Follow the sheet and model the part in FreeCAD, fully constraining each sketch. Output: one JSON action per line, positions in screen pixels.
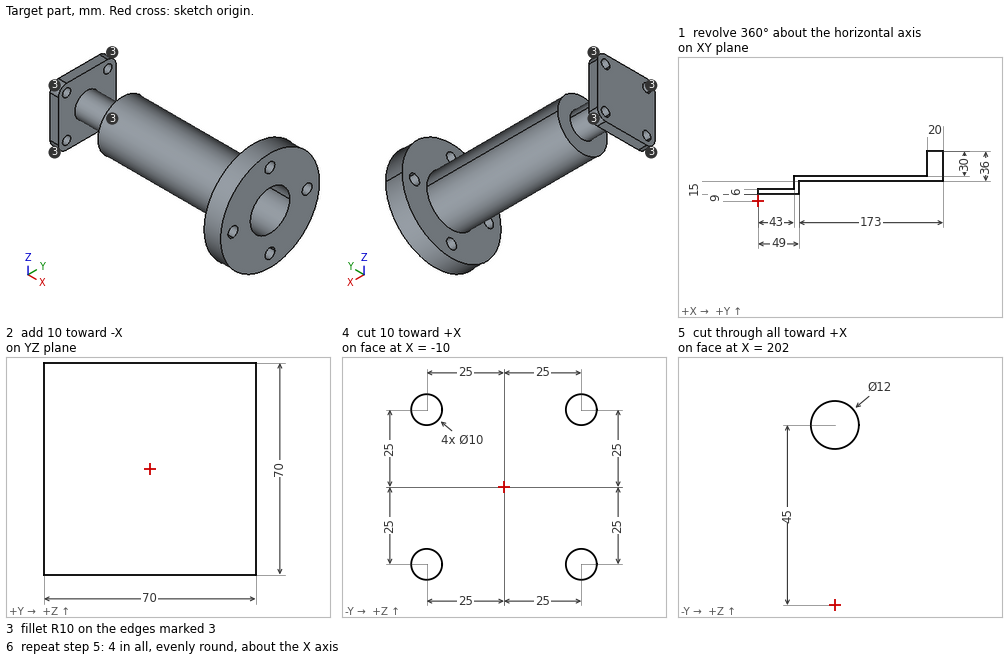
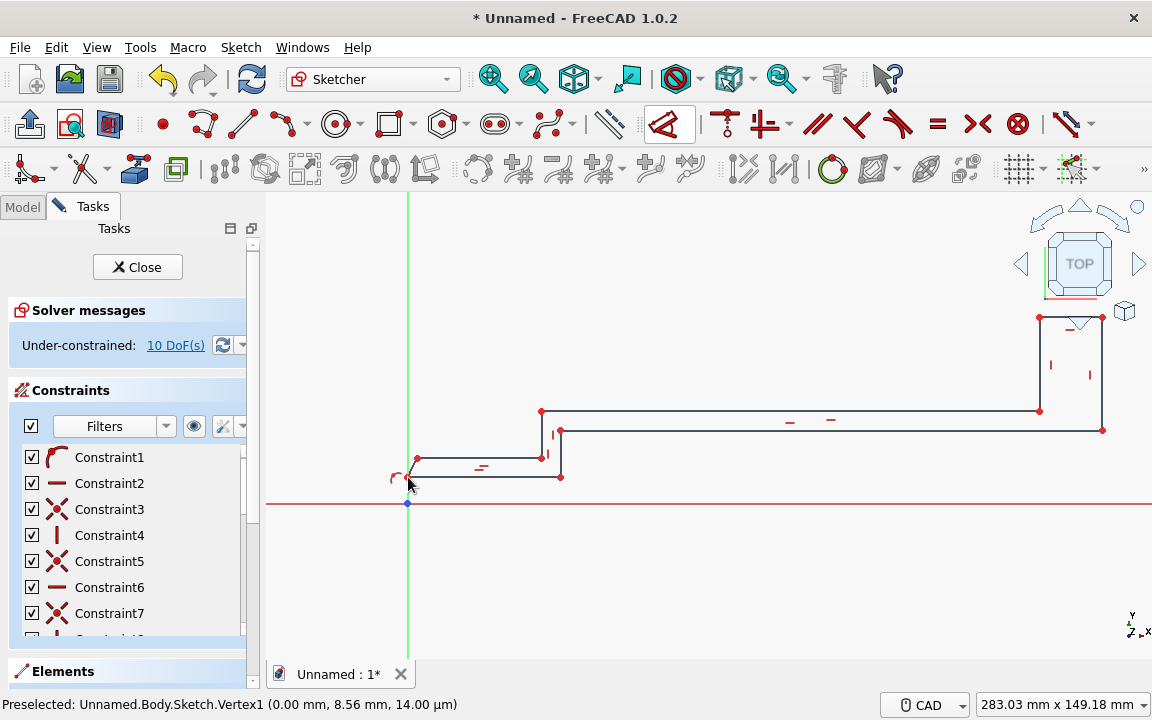
{"action": "scroll", "coordinate": [411, 470], "scroll_direction": "up", "scroll_amount": 4}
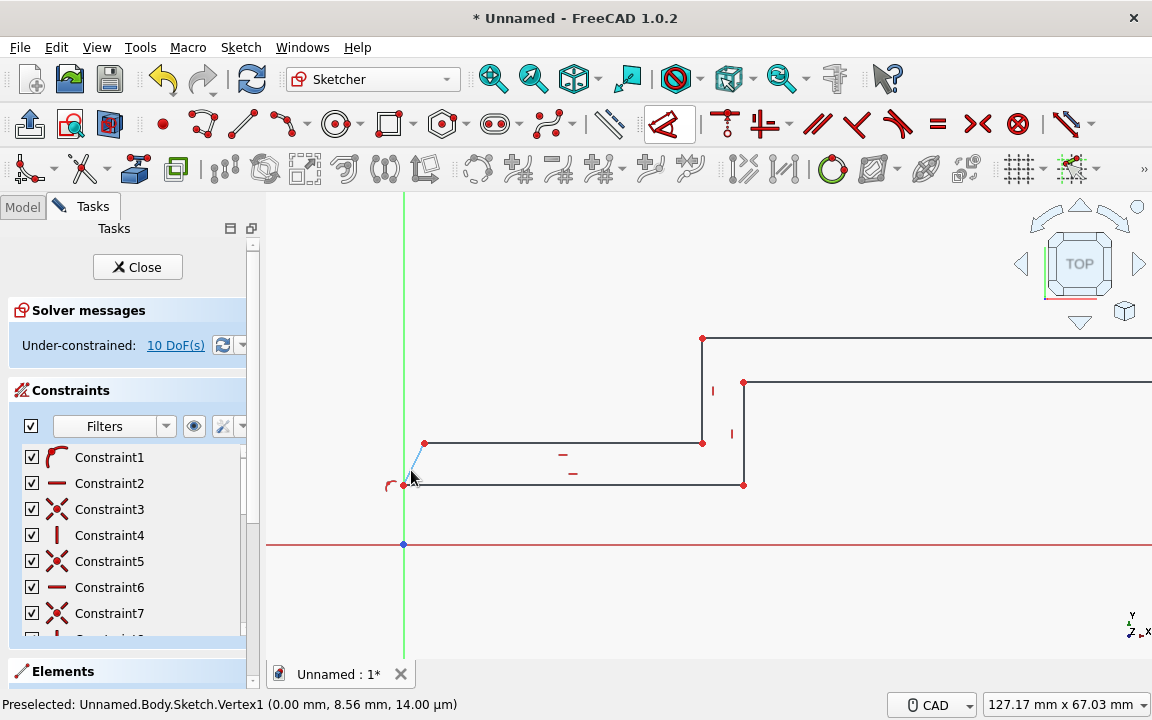
{"action": "left_click", "coordinate": [412, 468]}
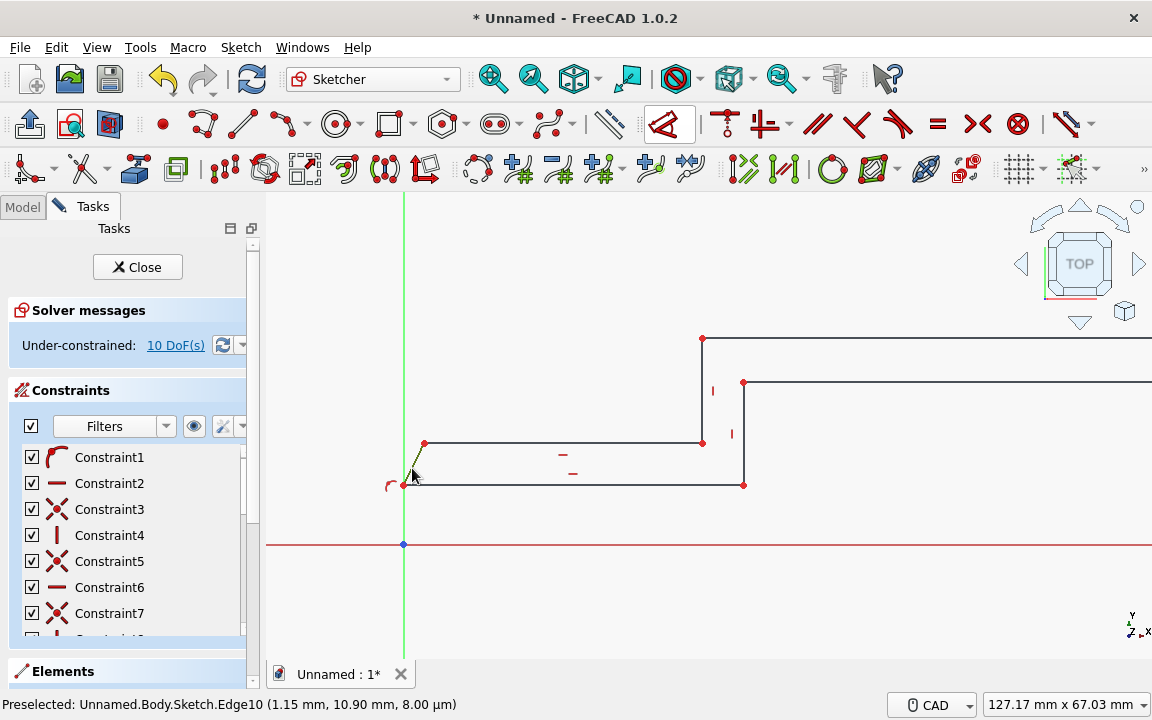
{"action": "key", "text": "v"}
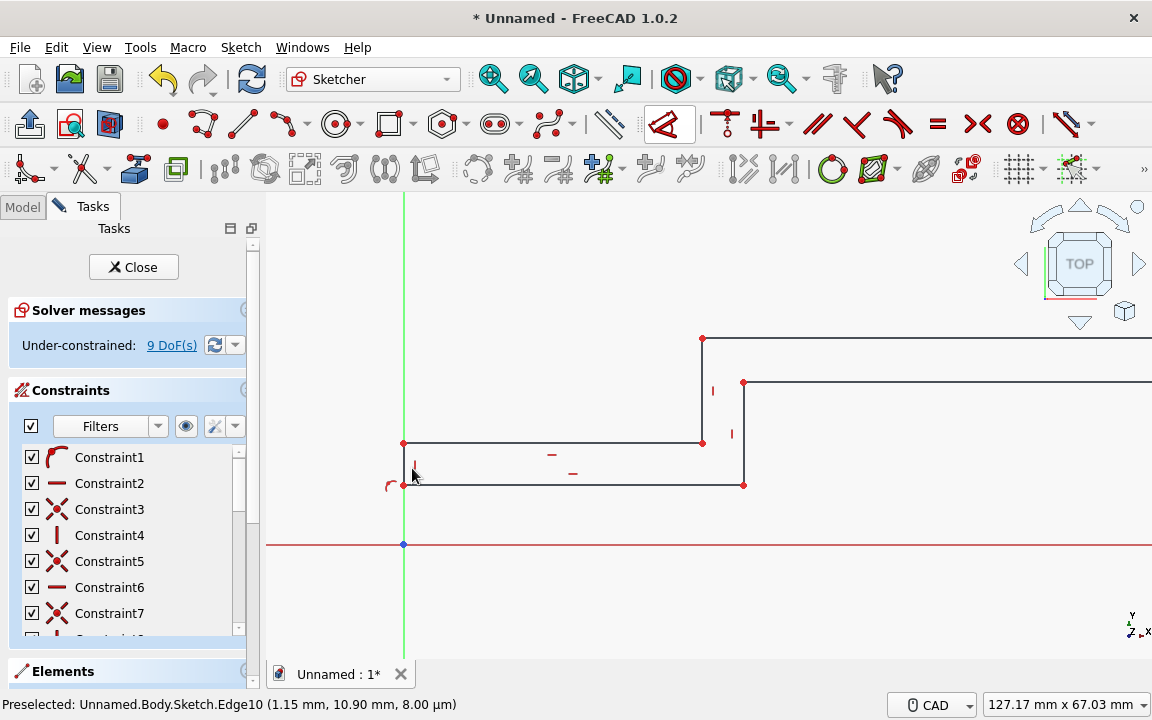
{"action": "left_click", "coordinate": [664, 124]}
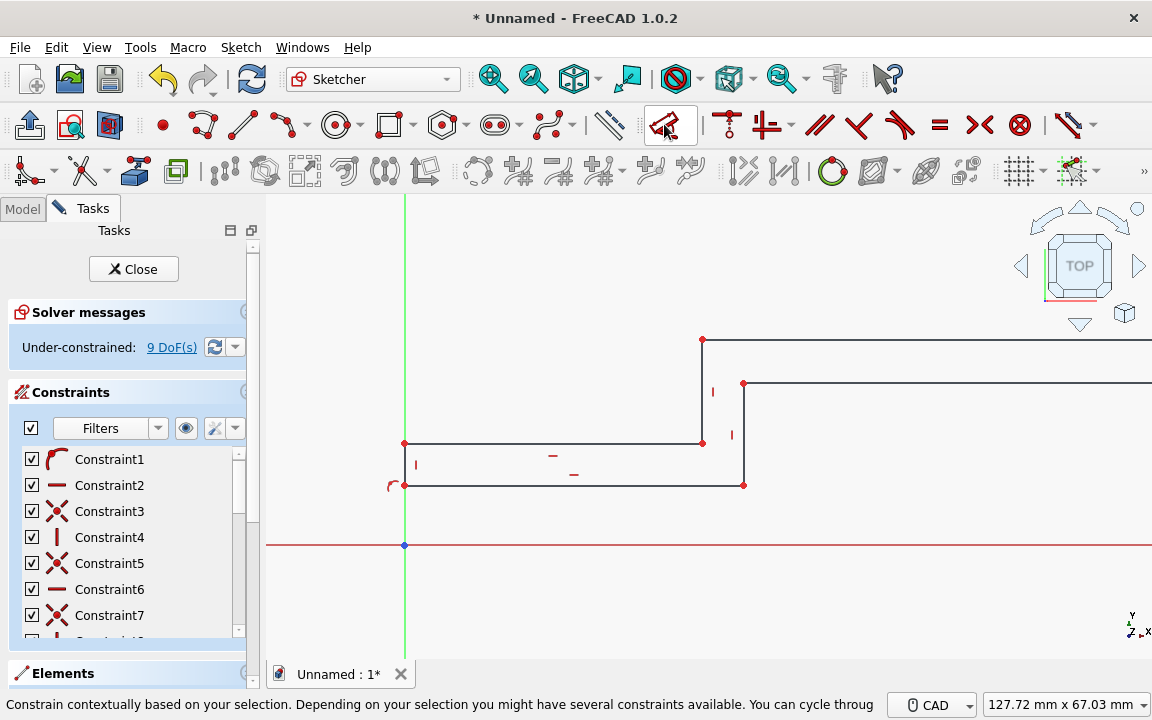
{"action": "left_click", "coordinate": [405, 457]}
{"action": "left_click", "coordinate": [371, 465]}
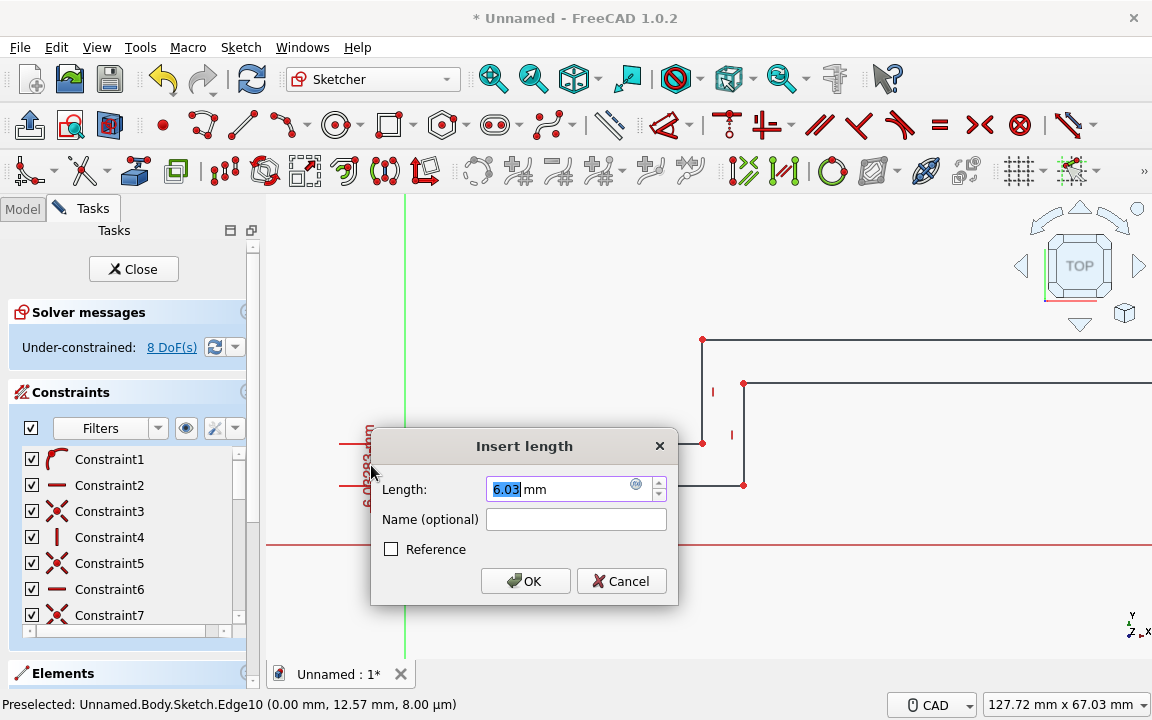
{"action": "type", "text": "6"}
{"action": "key", "text": "Return"}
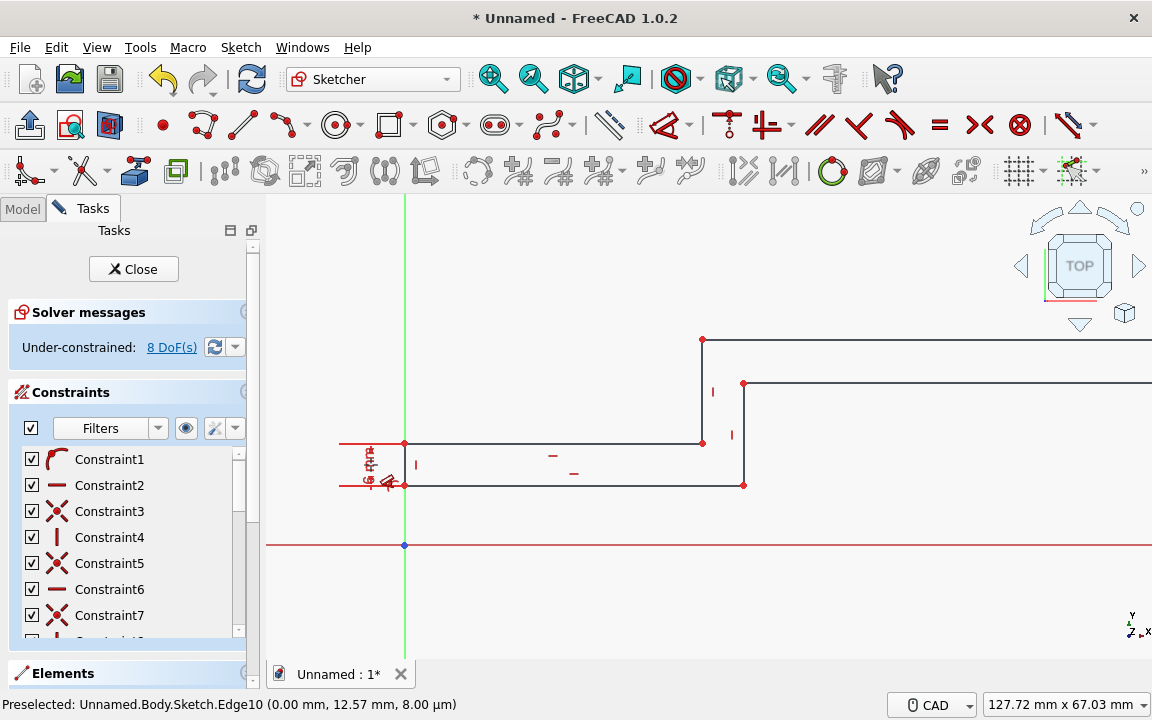
{"action": "left_click", "coordinate": [507, 486]}
{"action": "left_click", "coordinate": [574, 520]}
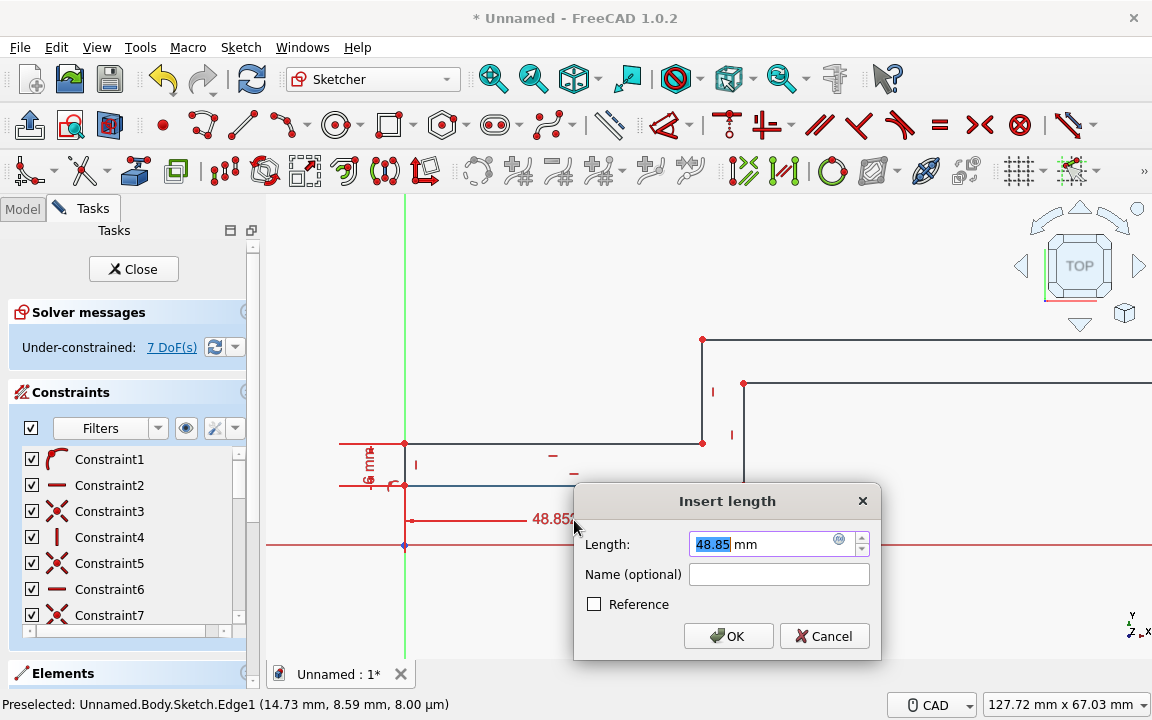
{"action": "type", "text": "49"}
{"action": "key", "text": "Return"}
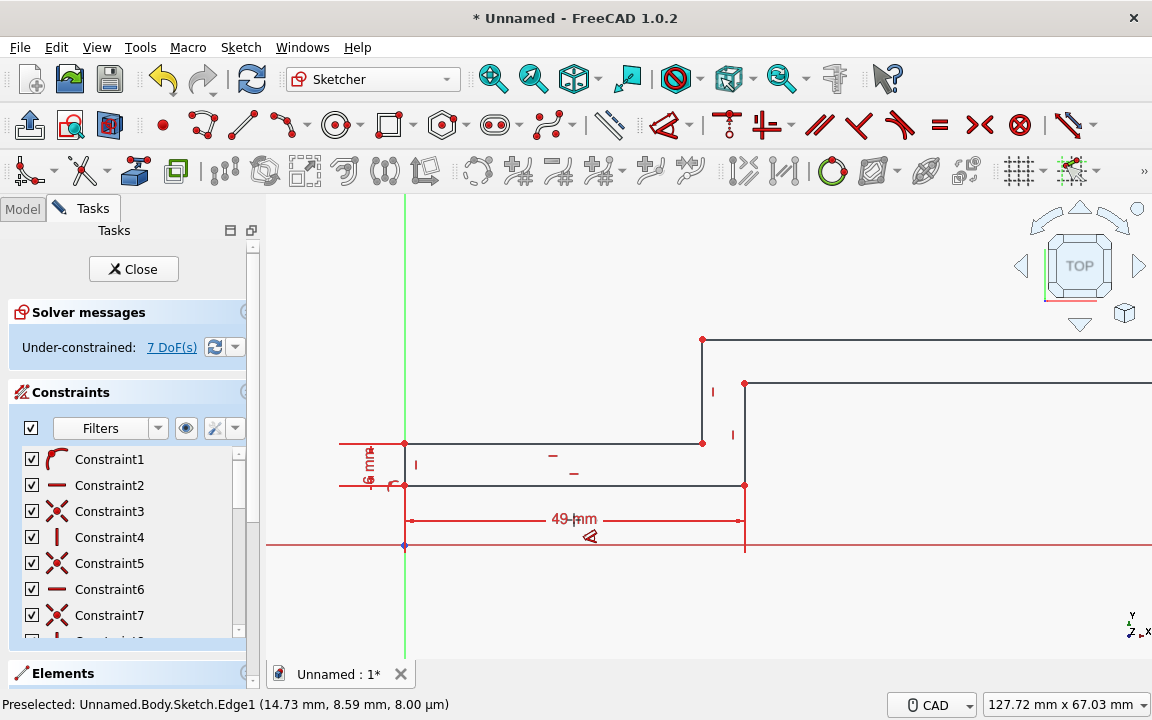
{"action": "left_click", "coordinate": [745, 455]}
{"action": "left_click", "coordinate": [711, 458]}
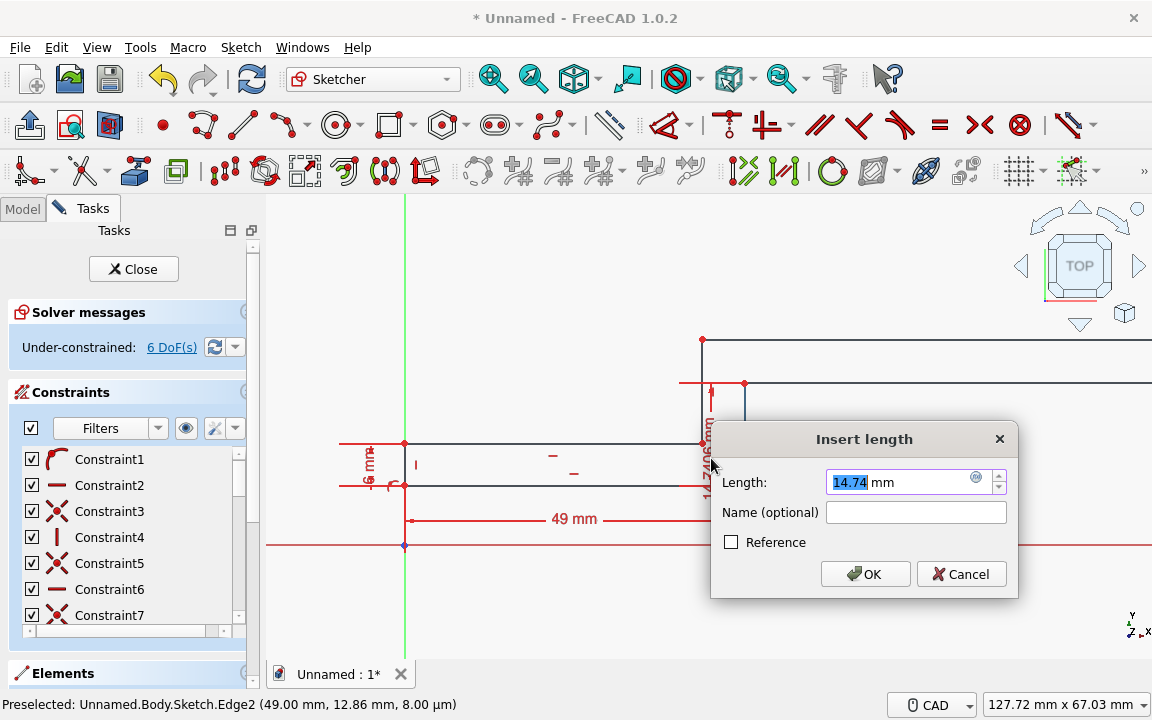
{"action": "type", "text": "15"}
{"action": "key", "text": "Return"}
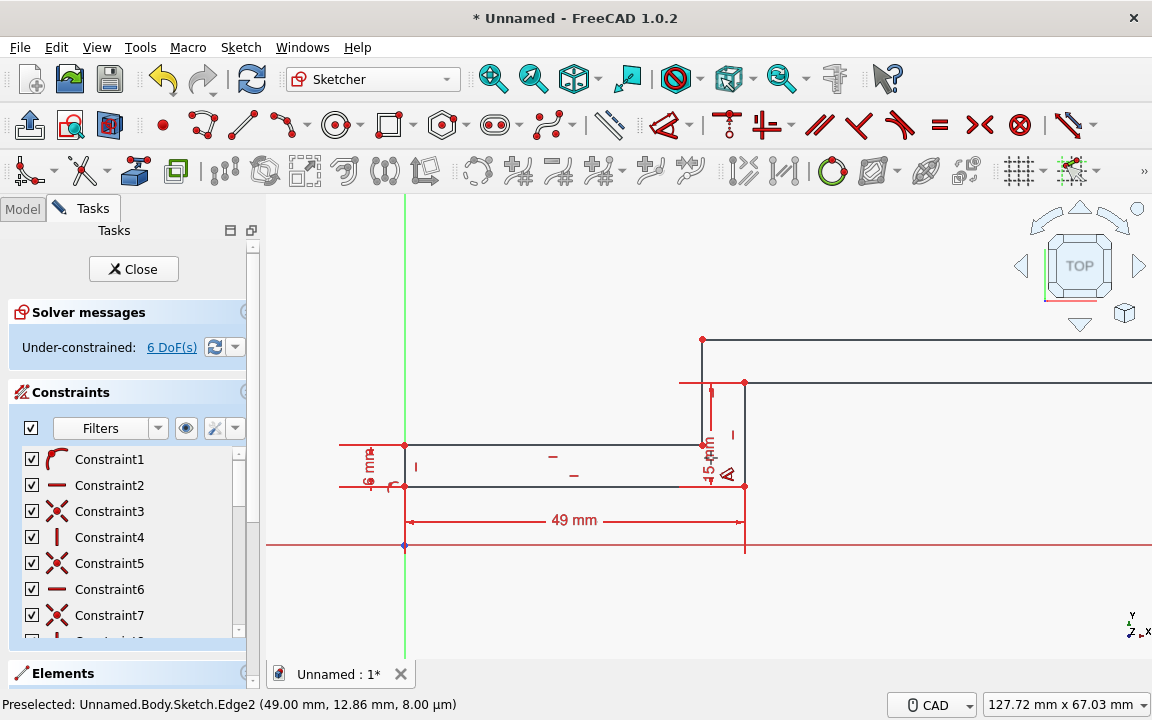
{"action": "scroll", "coordinate": [410, 465], "scroll_direction": "down", "scroll_amount": 6}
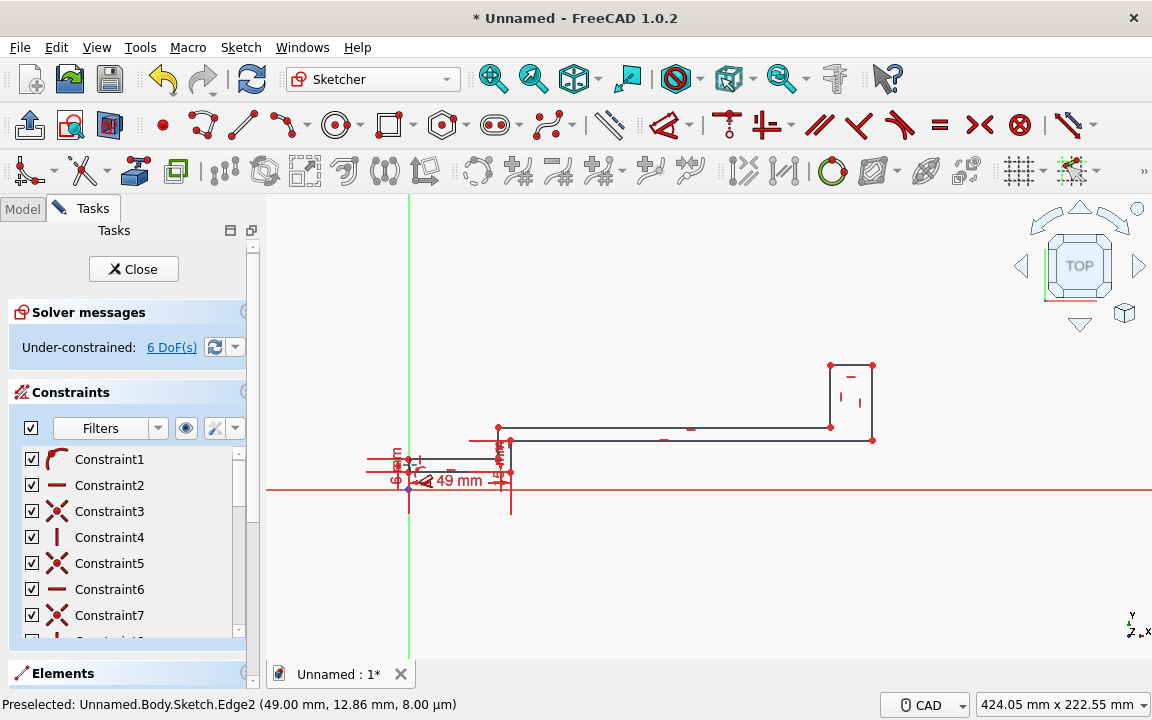
{"action": "left_click", "coordinate": [872, 418]}
{"action": "left_click", "coordinate": [906, 403]}